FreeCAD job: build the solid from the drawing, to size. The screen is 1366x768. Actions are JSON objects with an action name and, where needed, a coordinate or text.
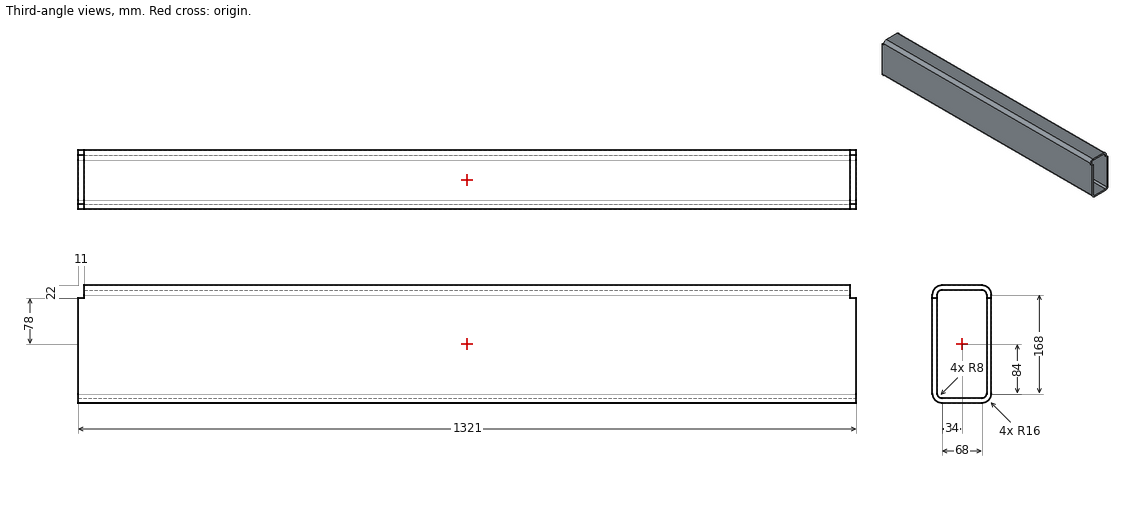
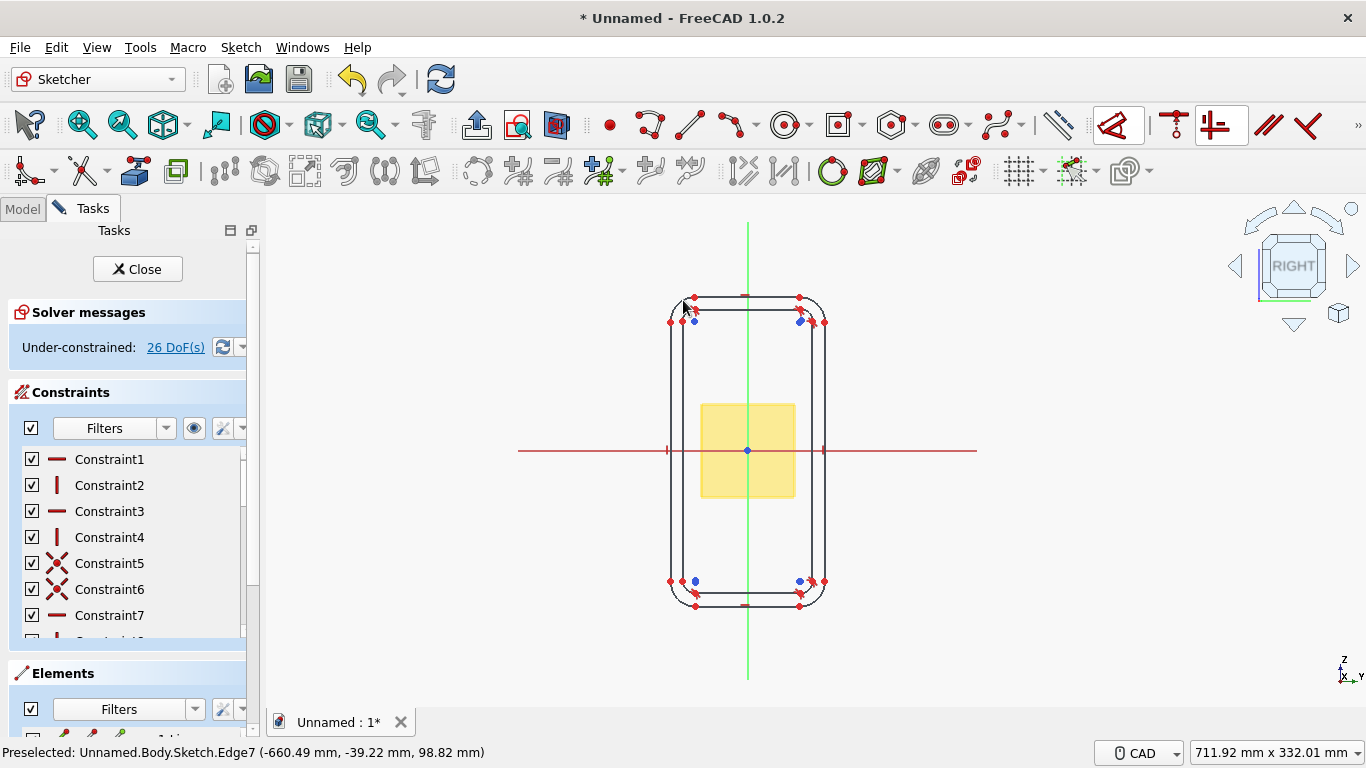
{"action": "left_click", "coordinate": [671, 400]}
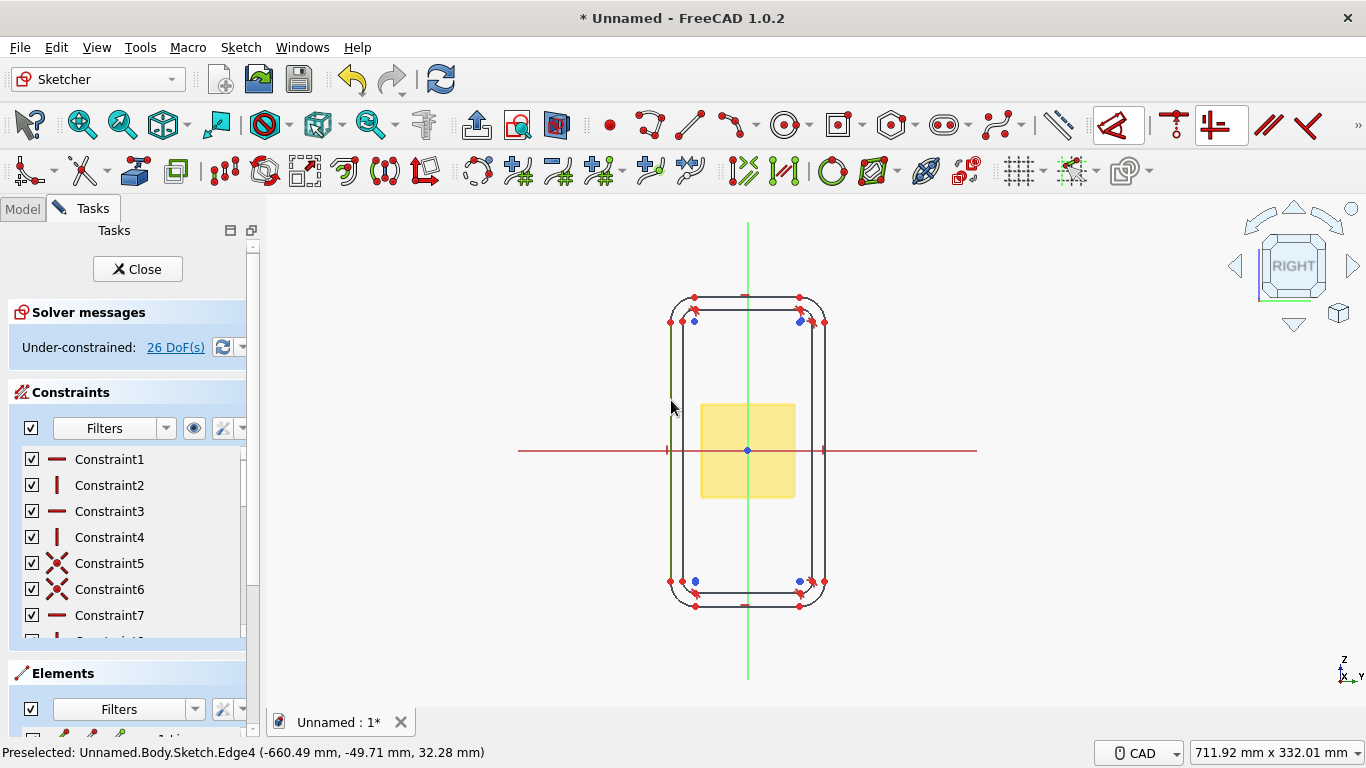
{"action": "left_click", "coordinate": [684, 300]}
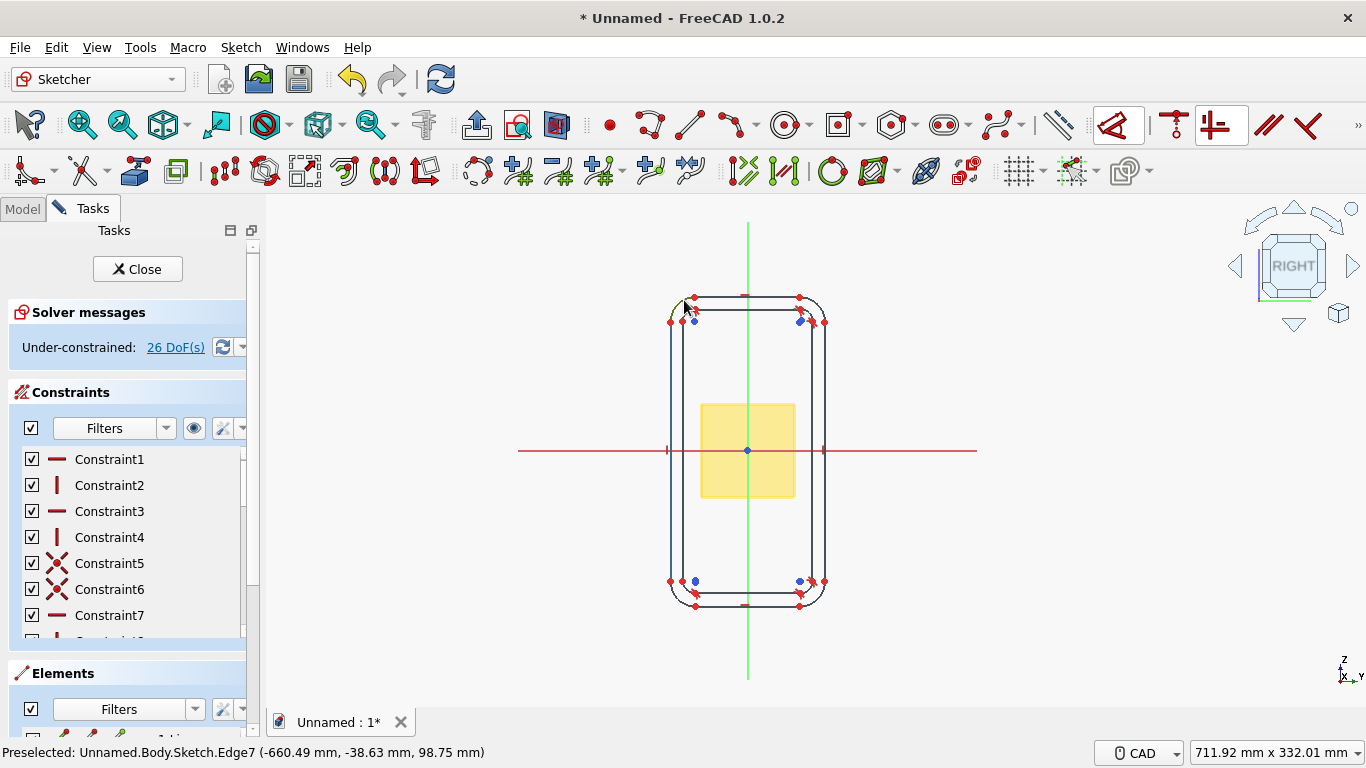
{"action": "key", "text": "t"}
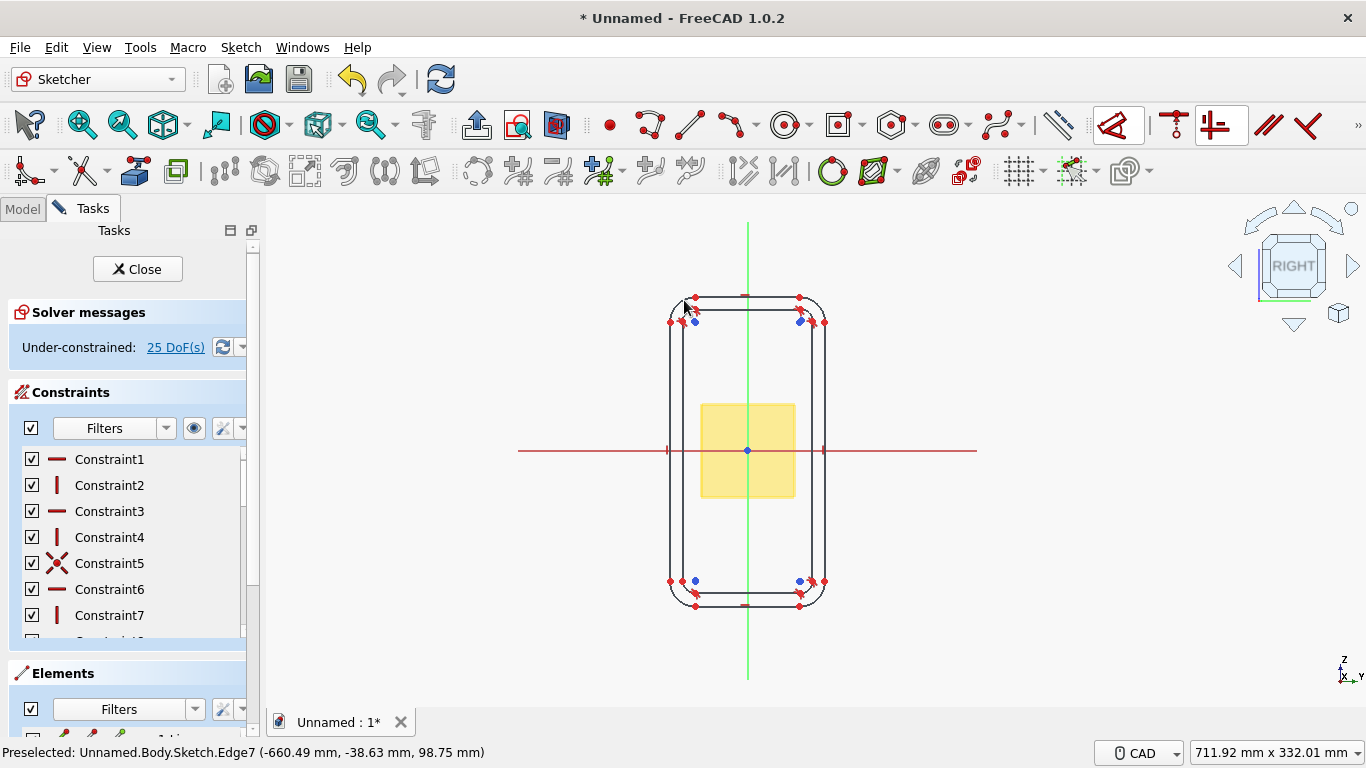
{"action": "left_click", "coordinate": [670, 400]}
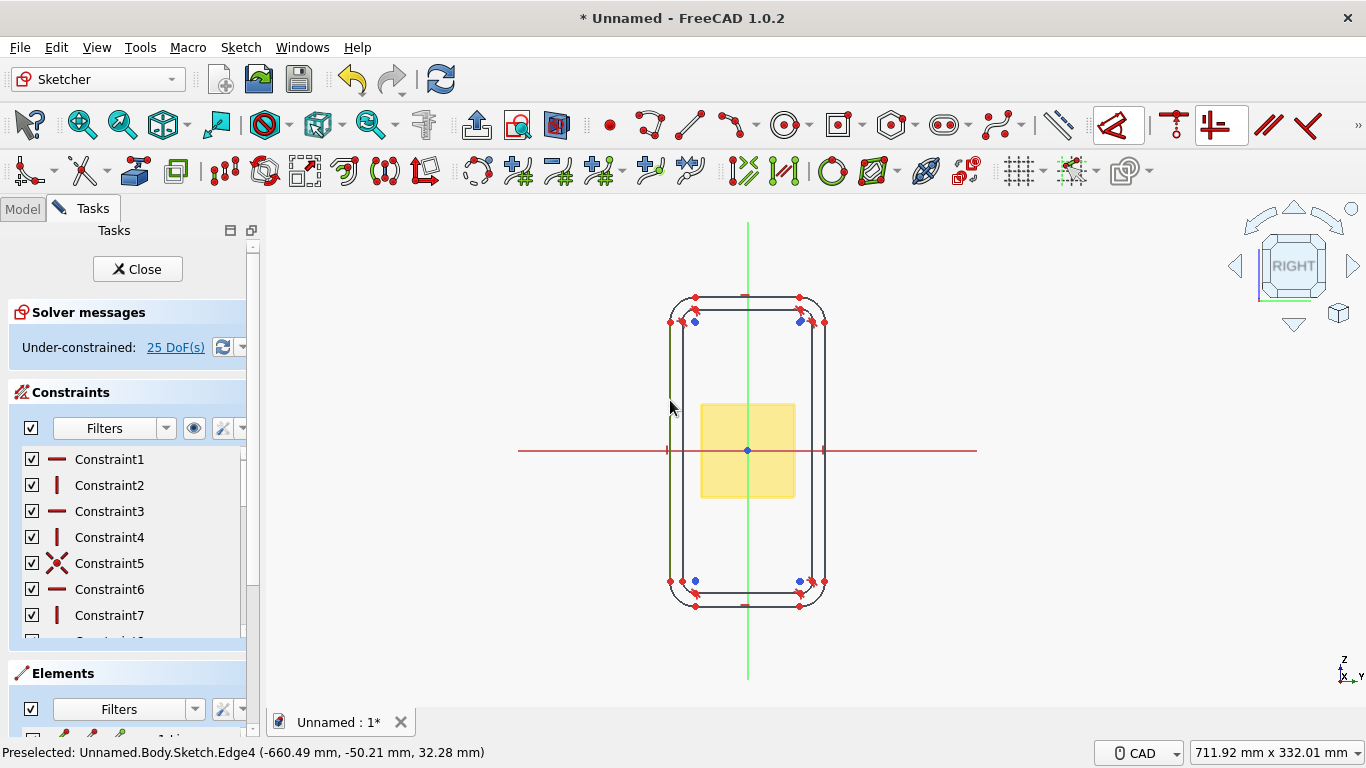
{"action": "left_click", "coordinate": [673, 593]}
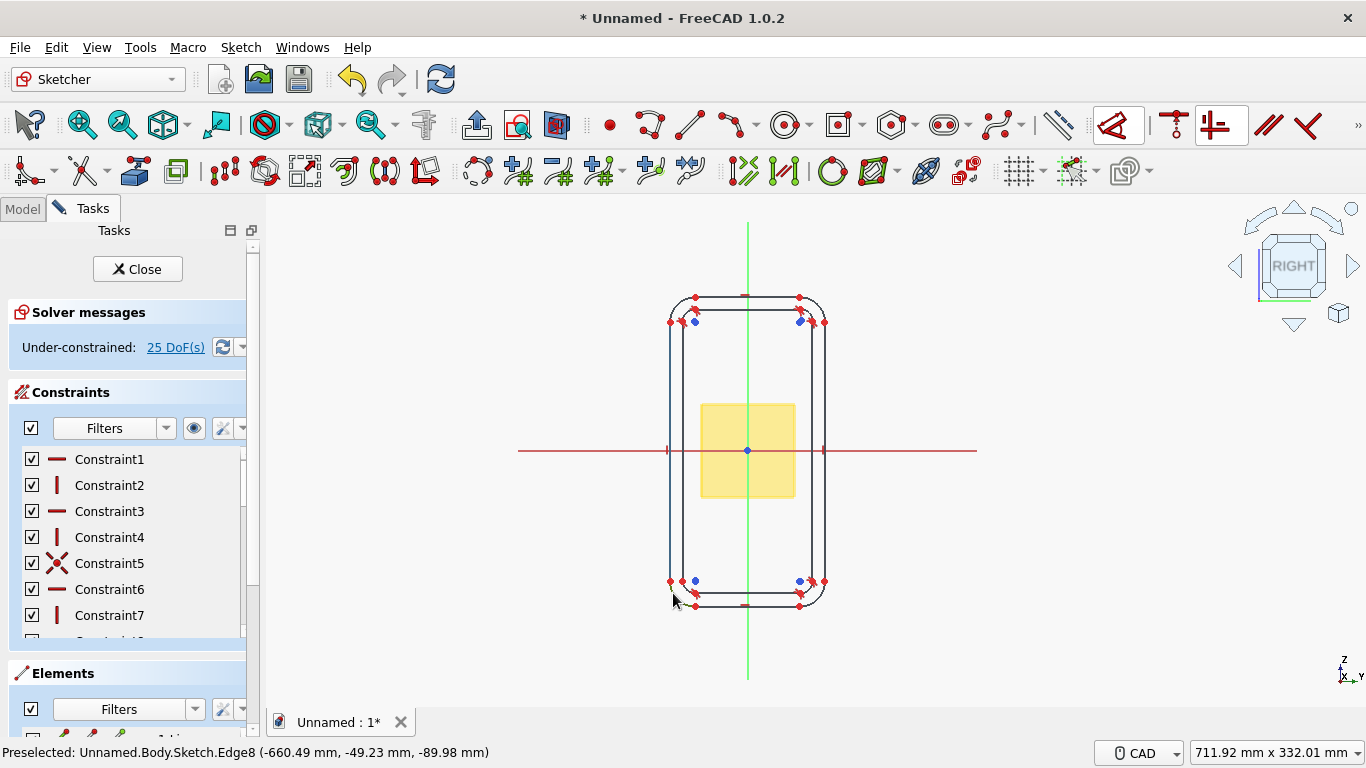
{"action": "key", "text": "t"}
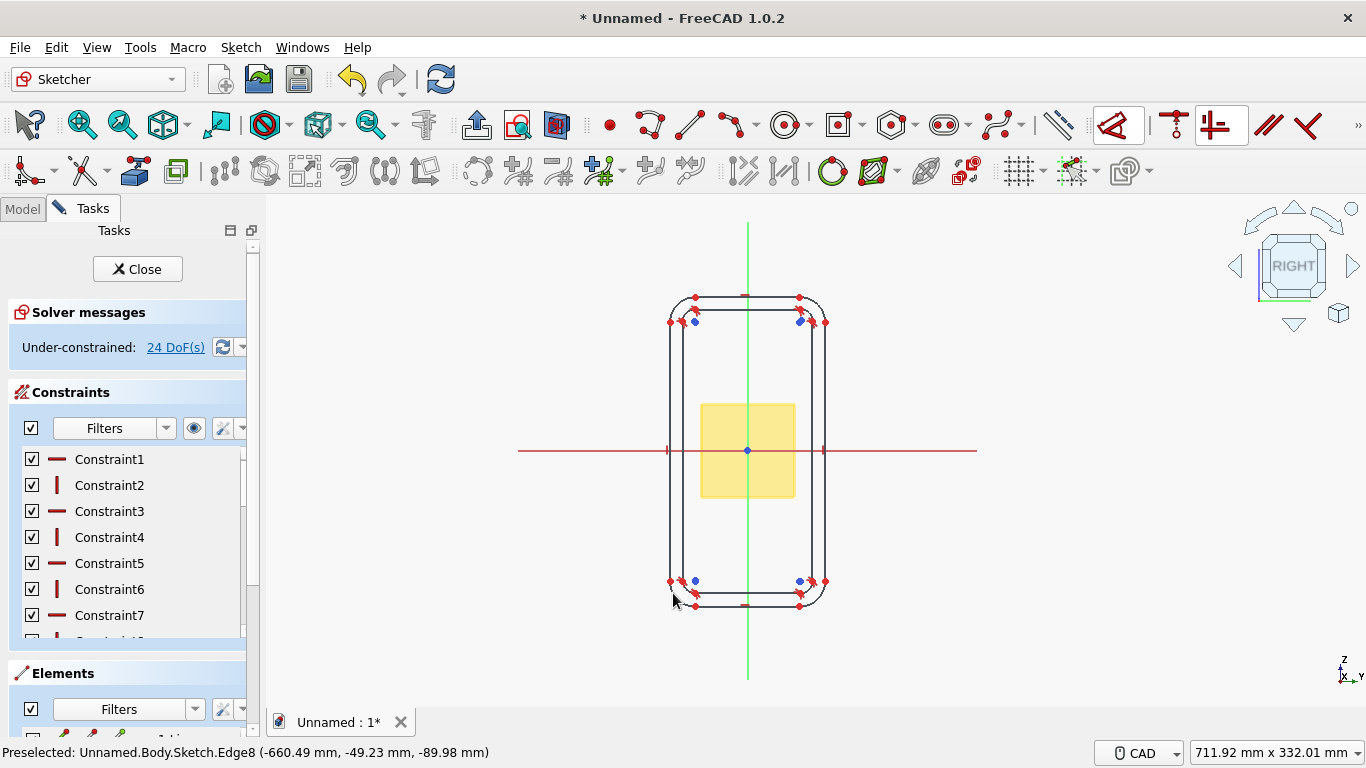
{"action": "left_click", "coordinate": [769, 593]}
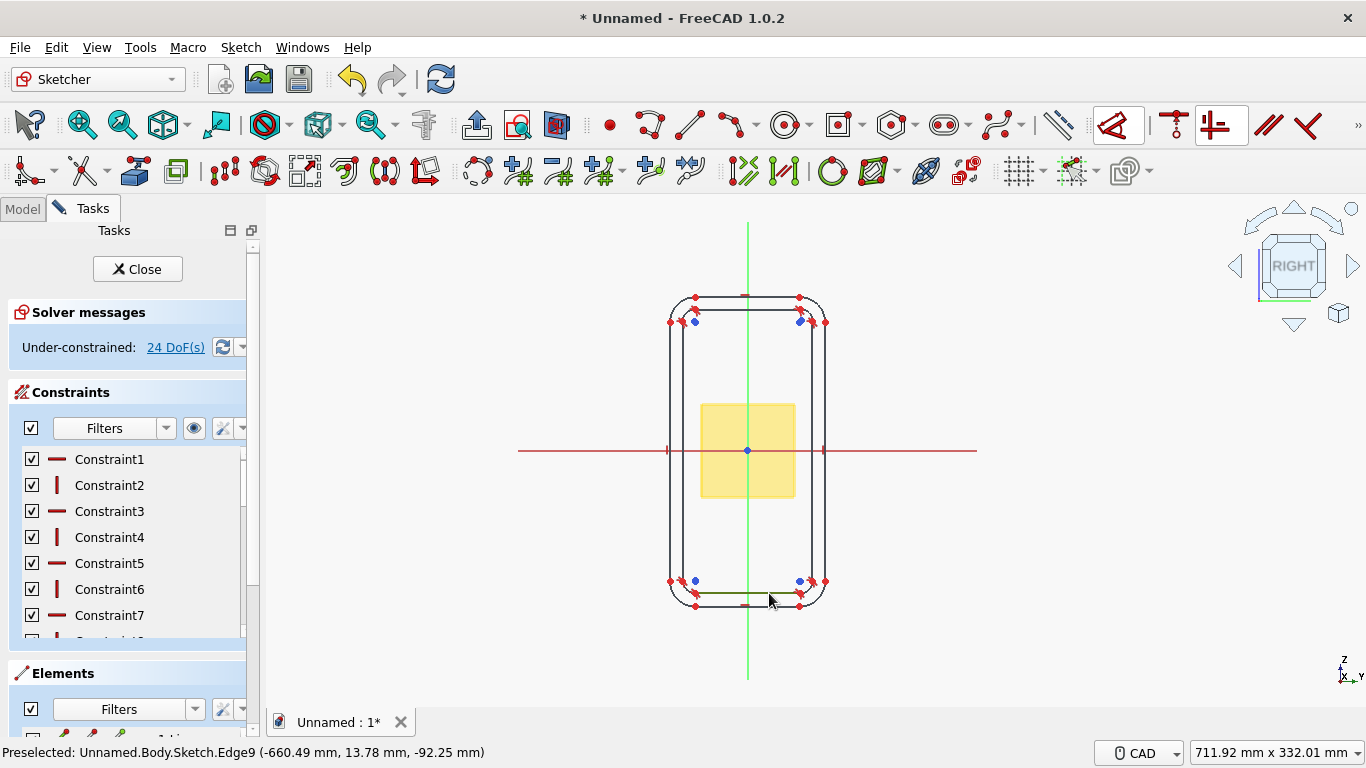
{"action": "scroll", "coordinate": [687, 590], "scroll_direction": "up", "scroll_amount": 2}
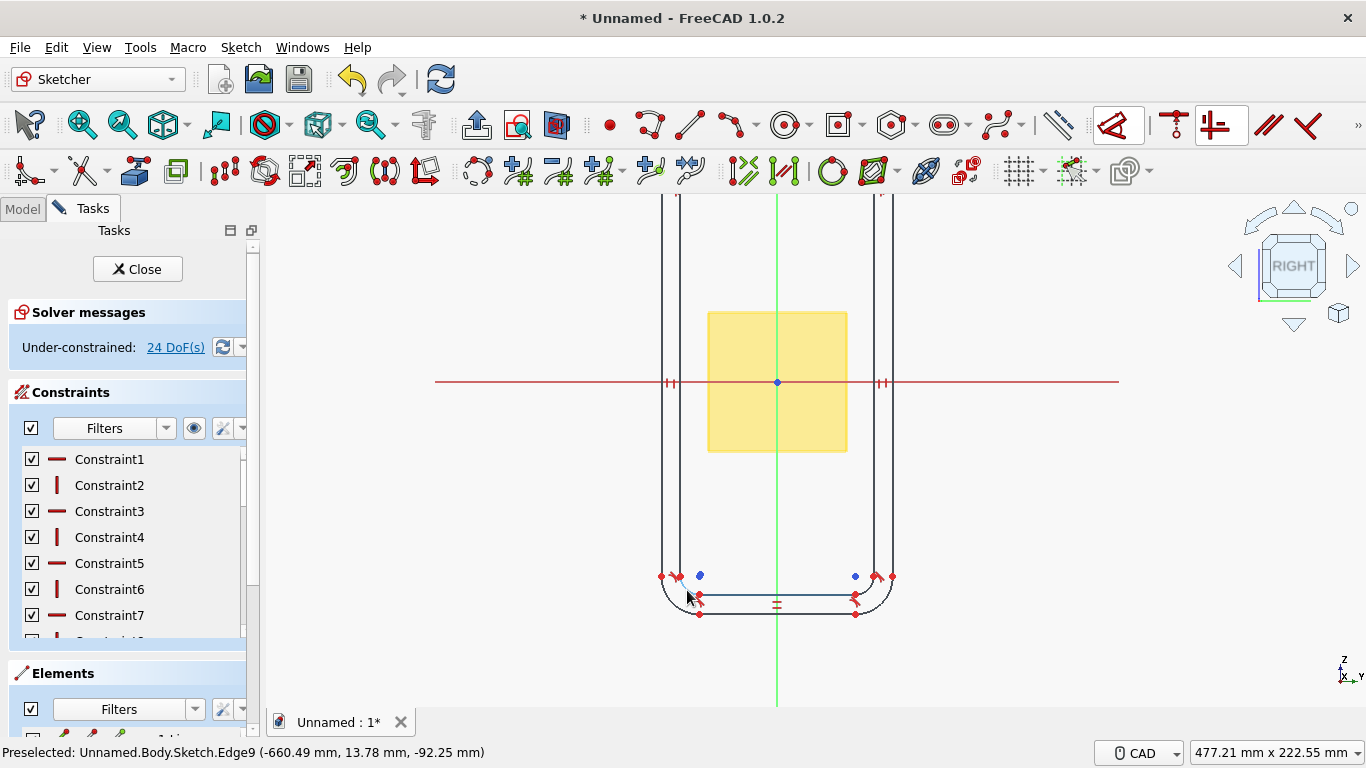
{"action": "left_click", "coordinate": [686, 589]}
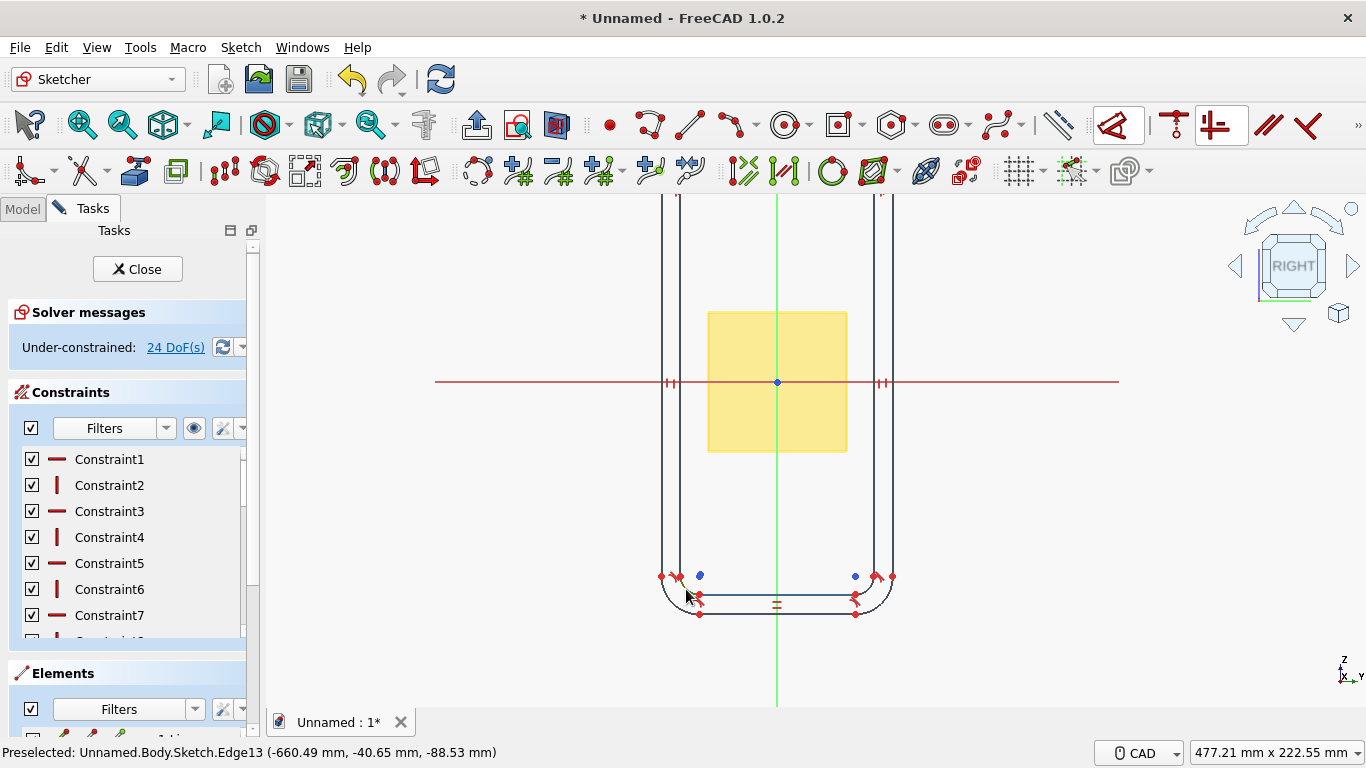
{"action": "key", "text": "t"}